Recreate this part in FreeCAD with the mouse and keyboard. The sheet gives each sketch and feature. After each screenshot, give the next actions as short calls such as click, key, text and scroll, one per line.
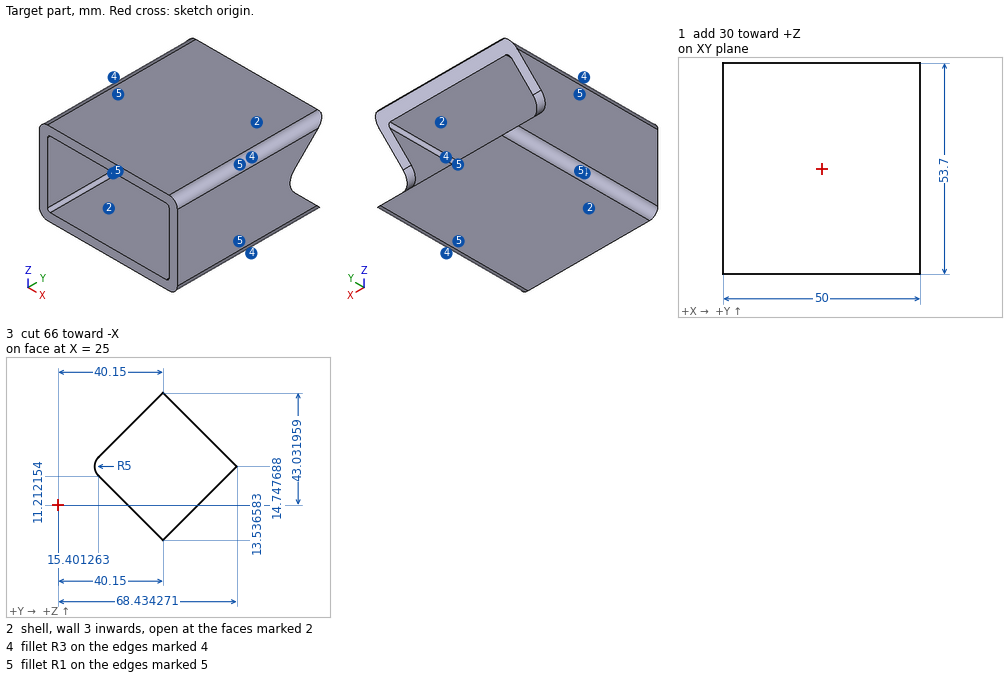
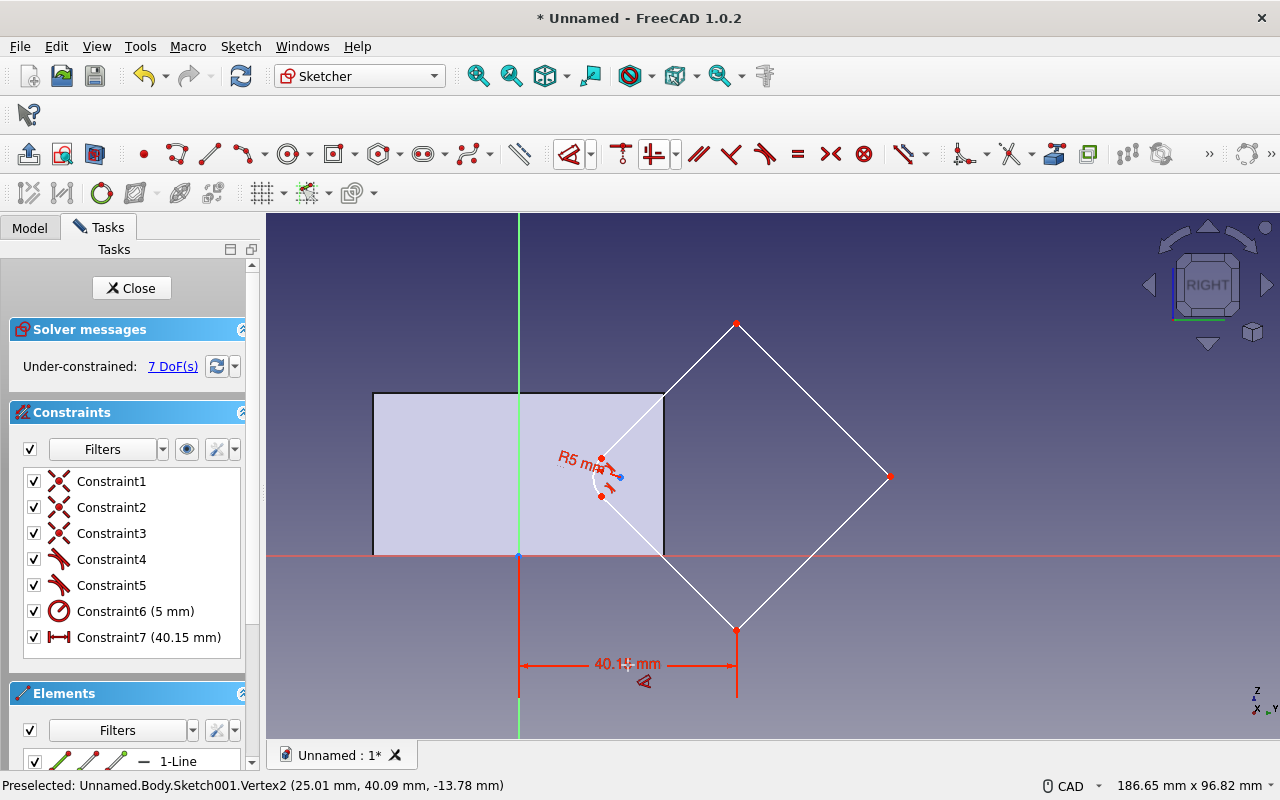
click(736, 323)
click(628, 289)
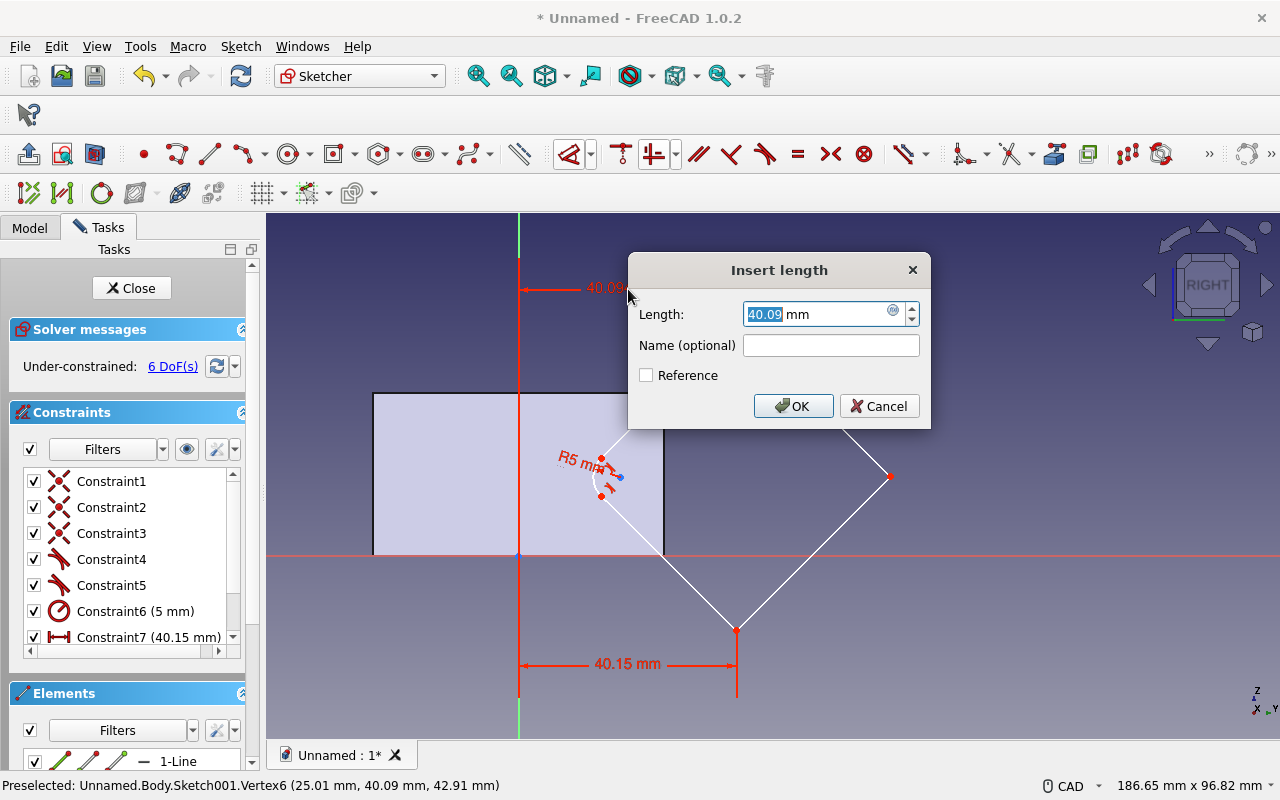
text(40.15)
key(Return)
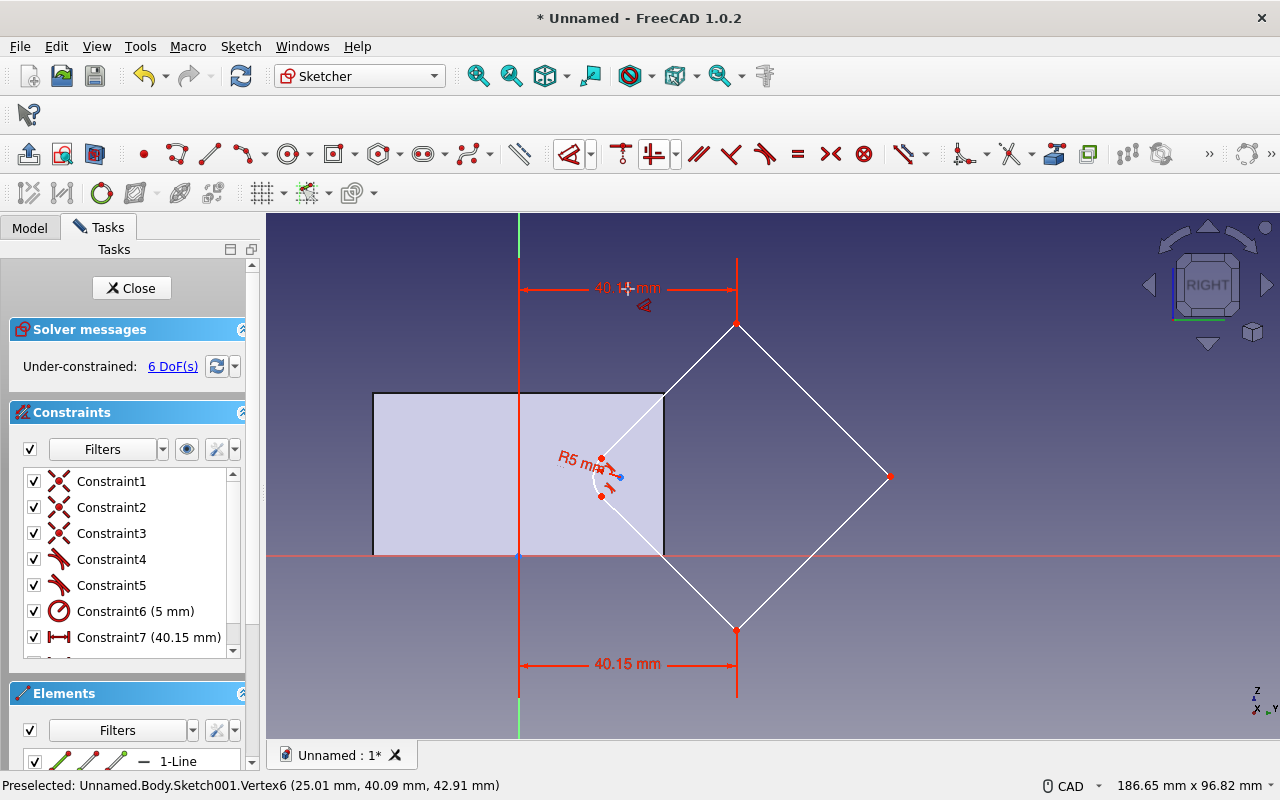
click(601, 497)
click(560, 590)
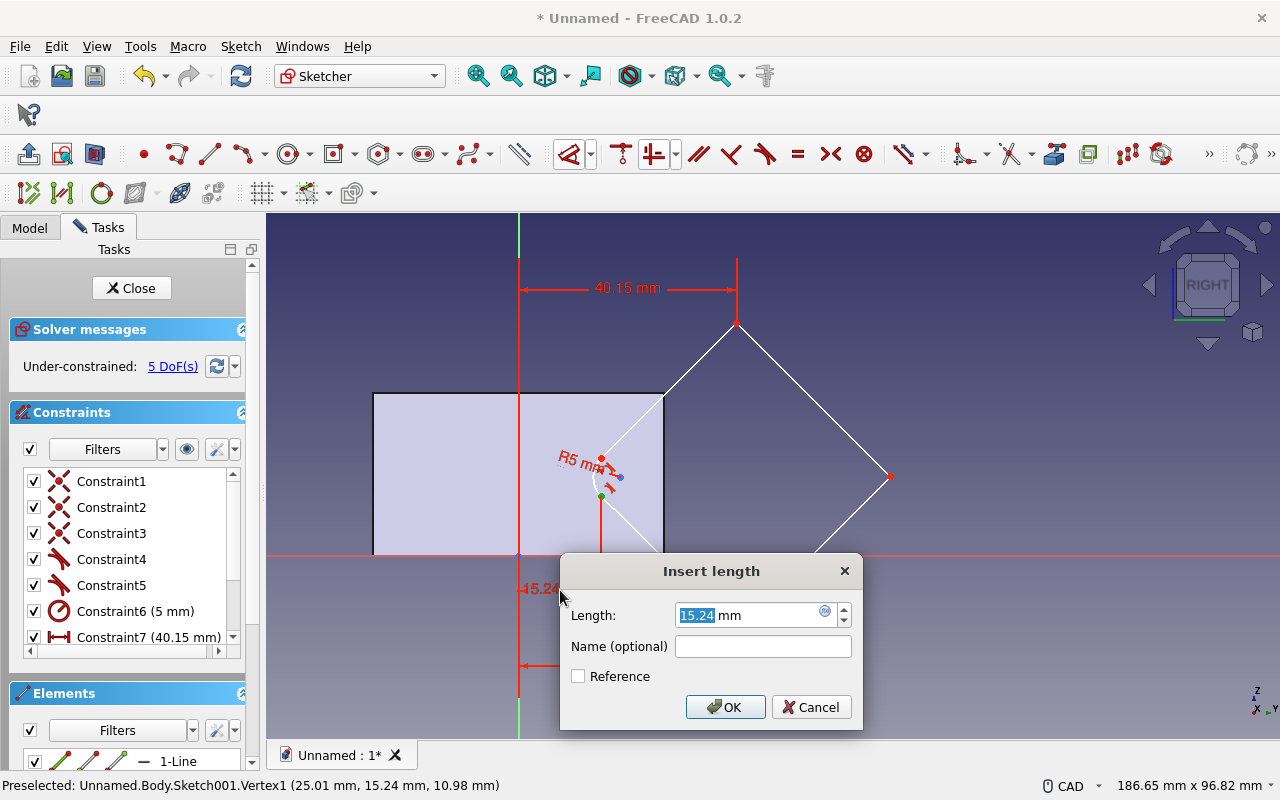
text(15.401263)
key(Return)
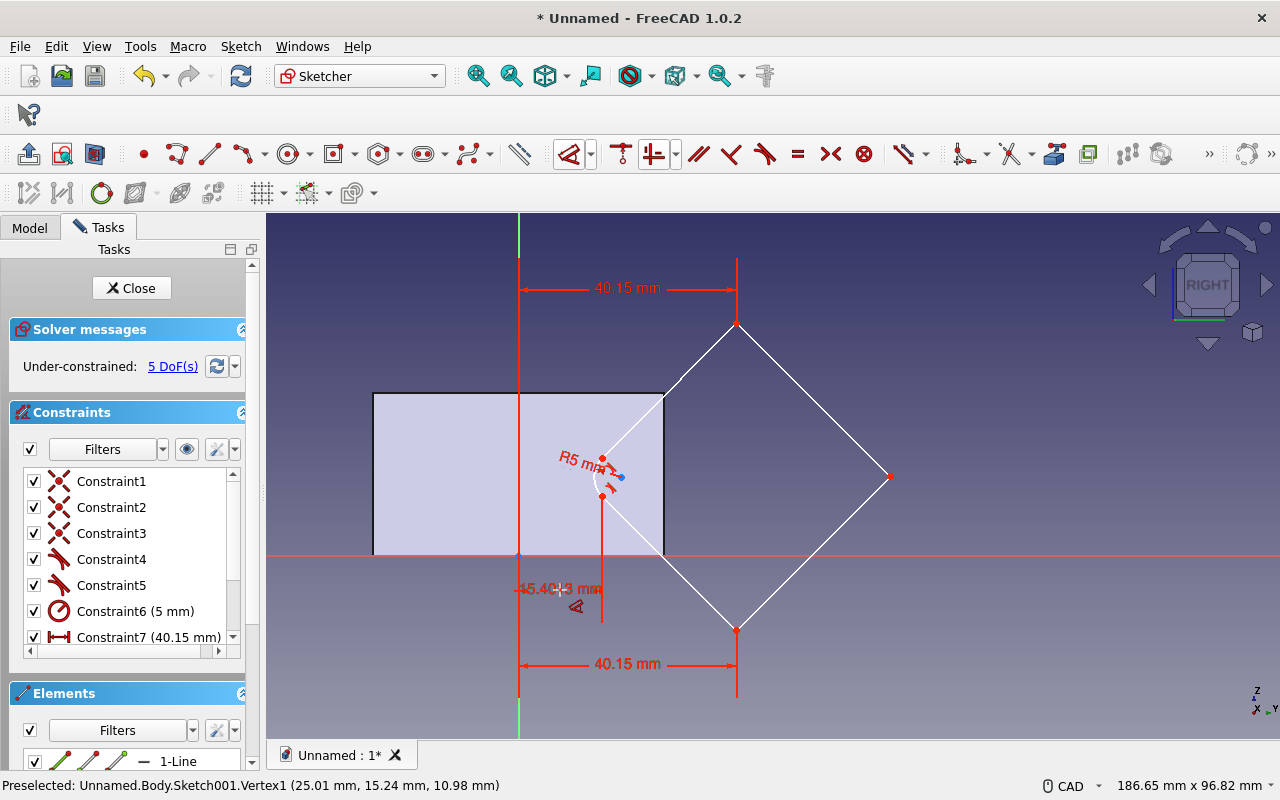
click(602, 497)
click(485, 526)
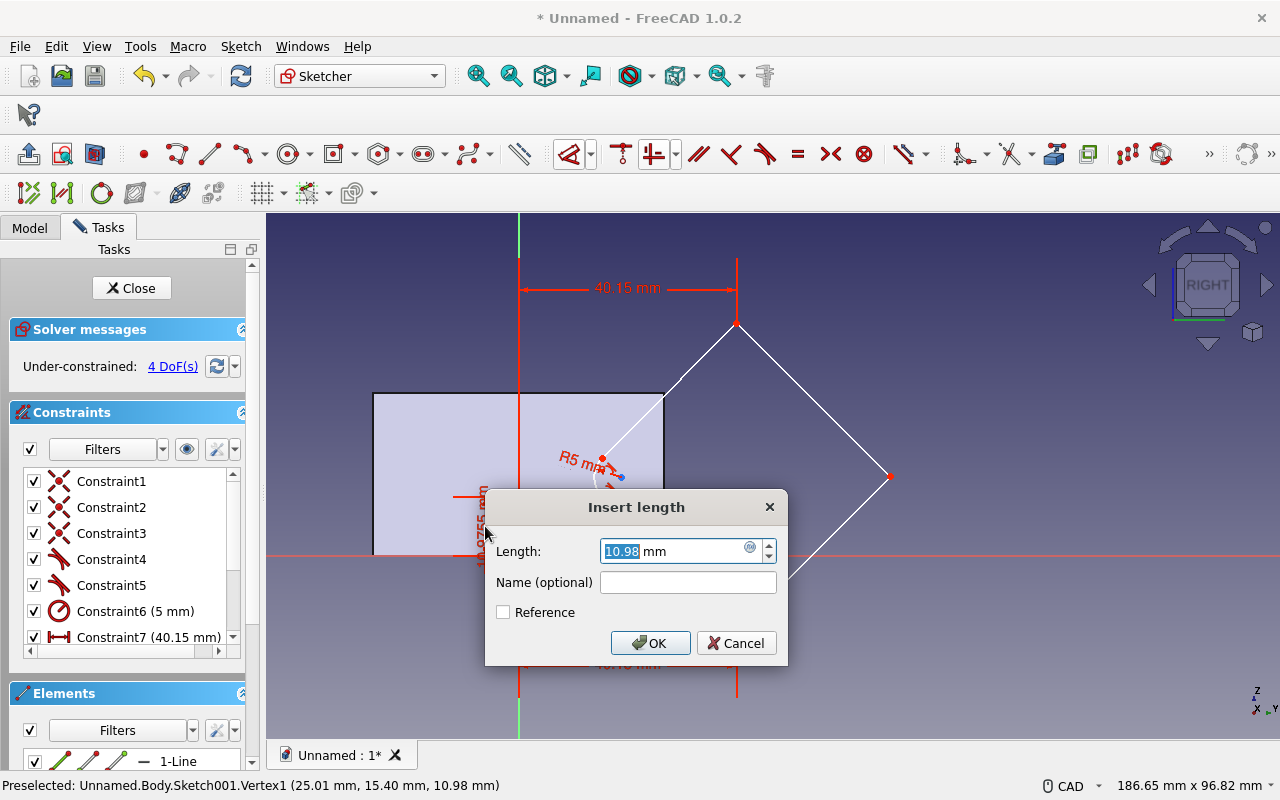
text(11.212154)
key(Return)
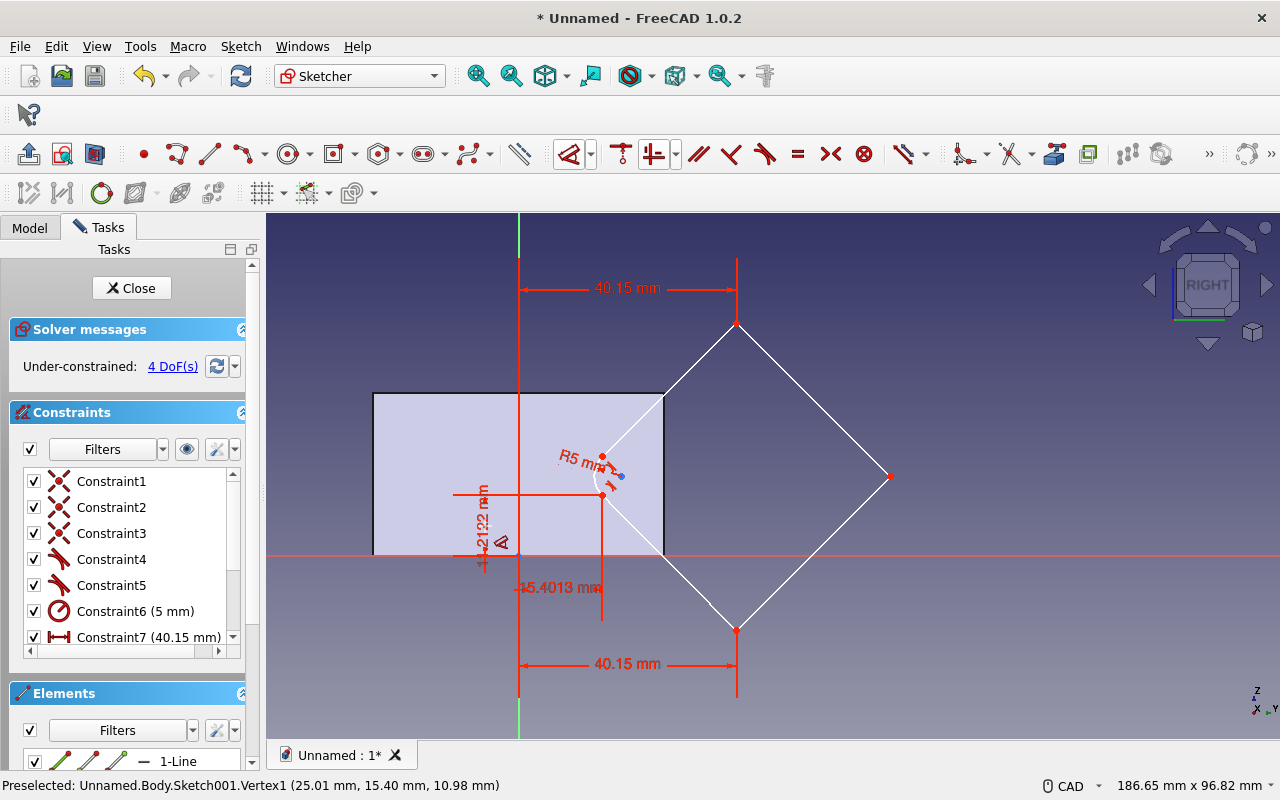
click(737, 631)
click(485, 594)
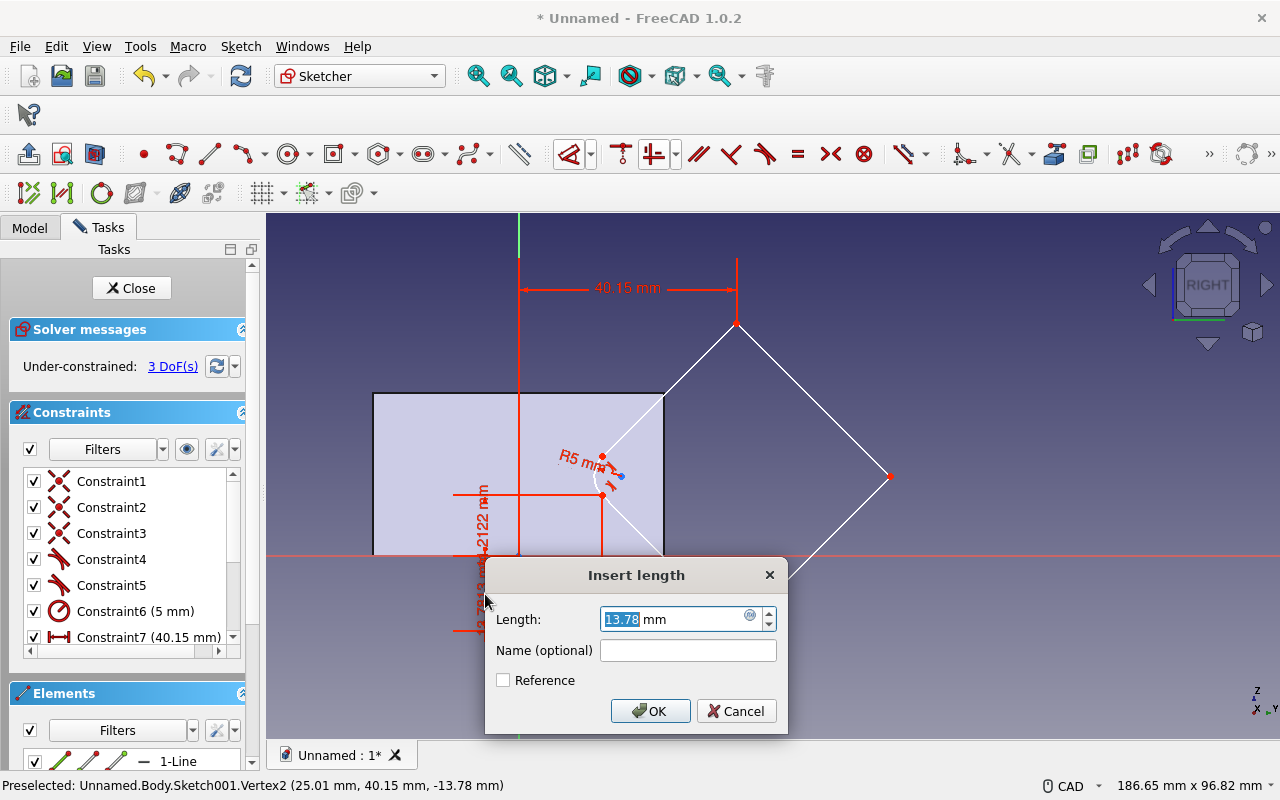
text(13.536583)
key(Return)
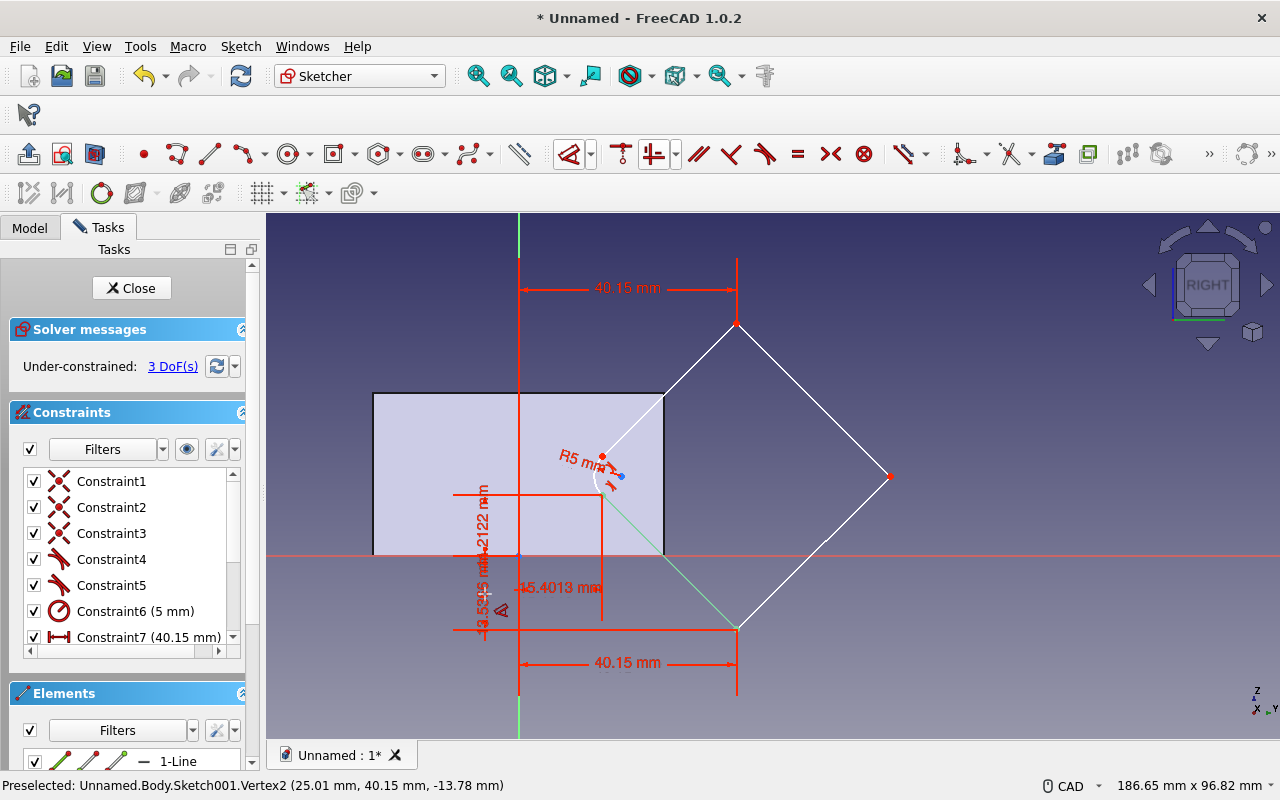
click(890, 477)
click(835, 590)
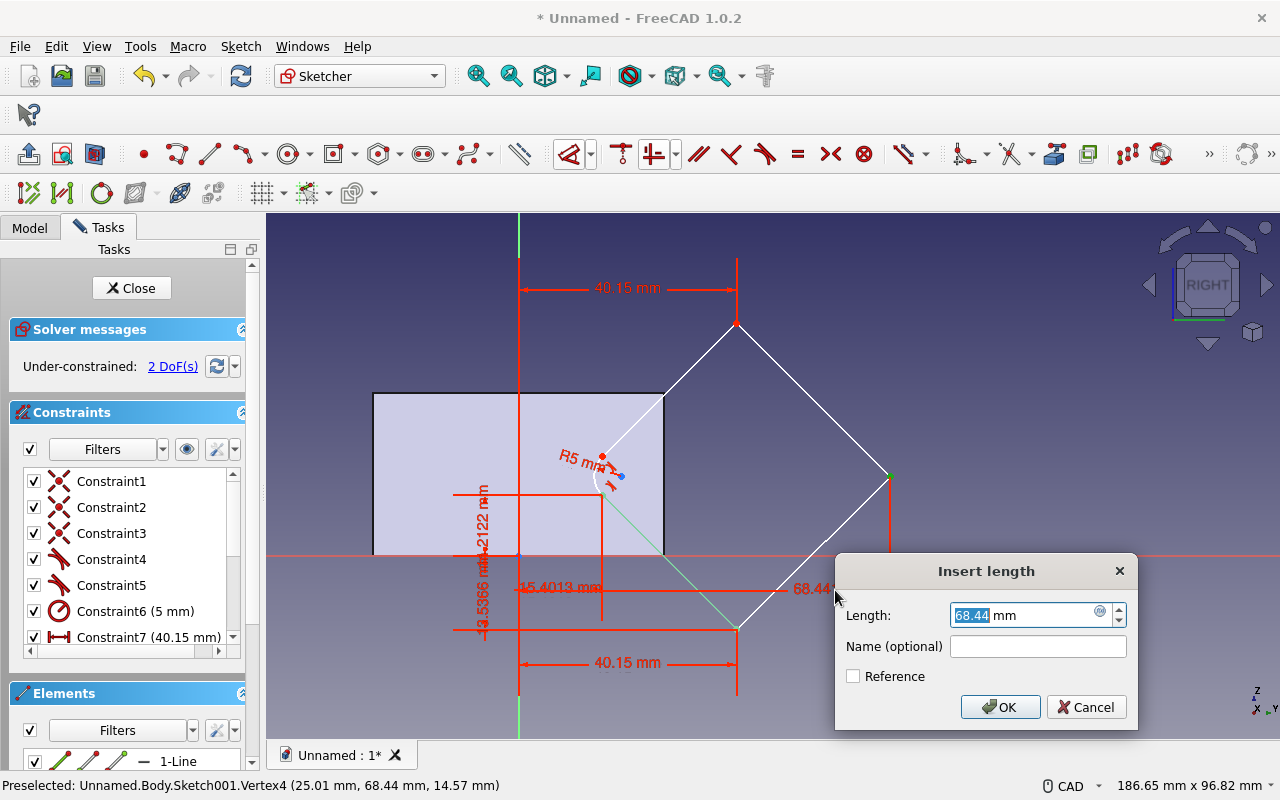
text(68.434271)
key(Return)